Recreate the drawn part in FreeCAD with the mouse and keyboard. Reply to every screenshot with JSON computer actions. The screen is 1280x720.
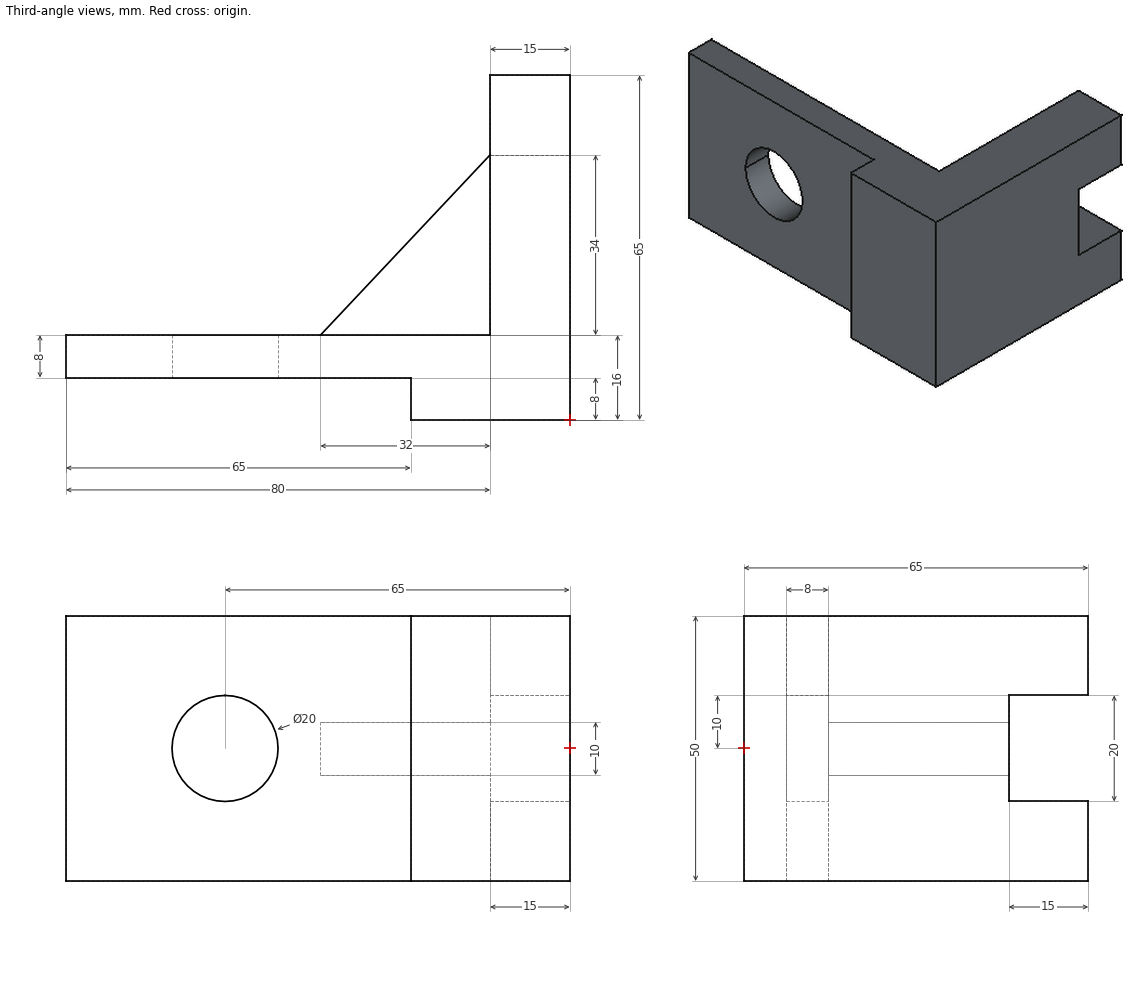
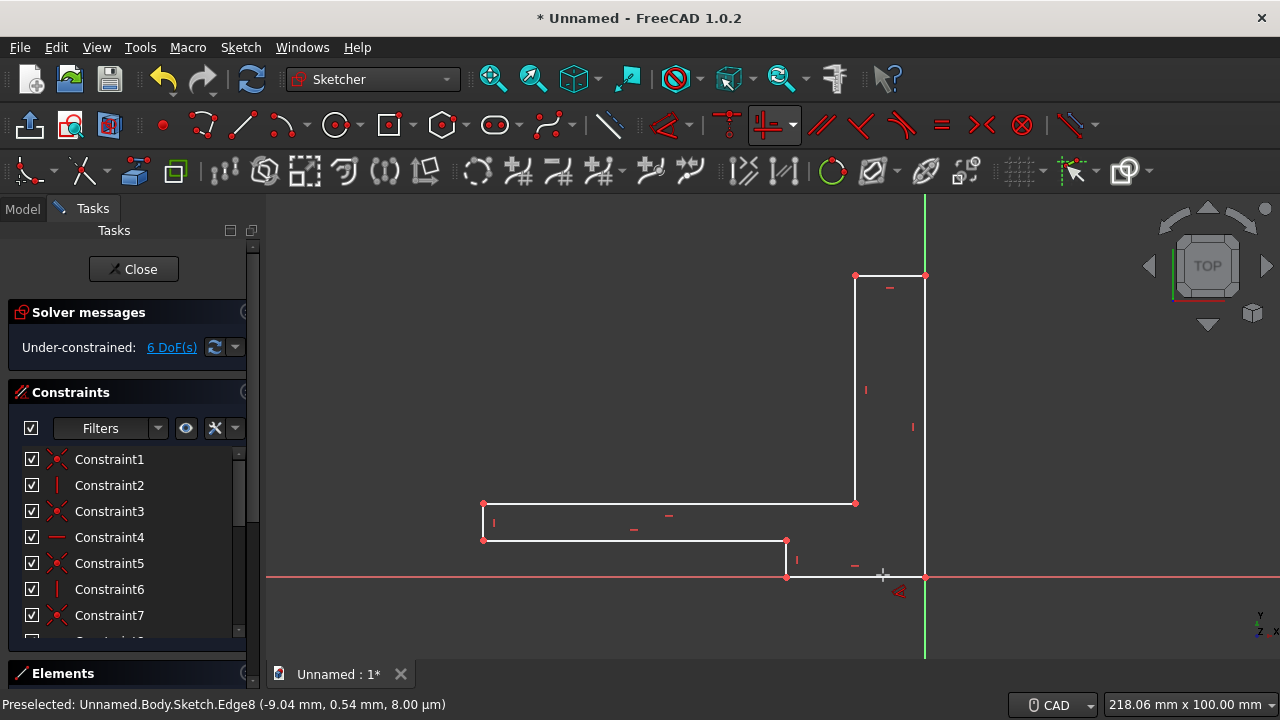
{"action": "scroll", "coordinate": [483, 515], "scroll_direction": "up", "scroll_amount": 2}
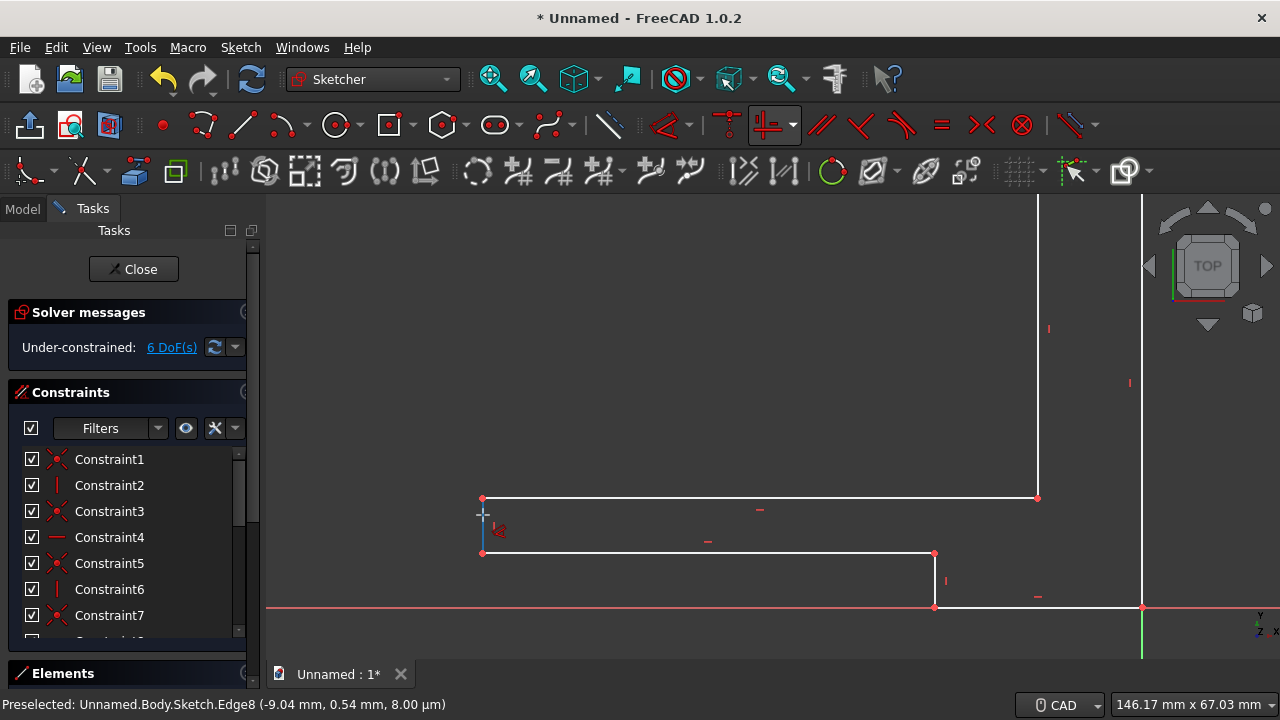
{"action": "left_click", "coordinate": [483, 515]}
{"action": "left_click", "coordinate": [449, 526]}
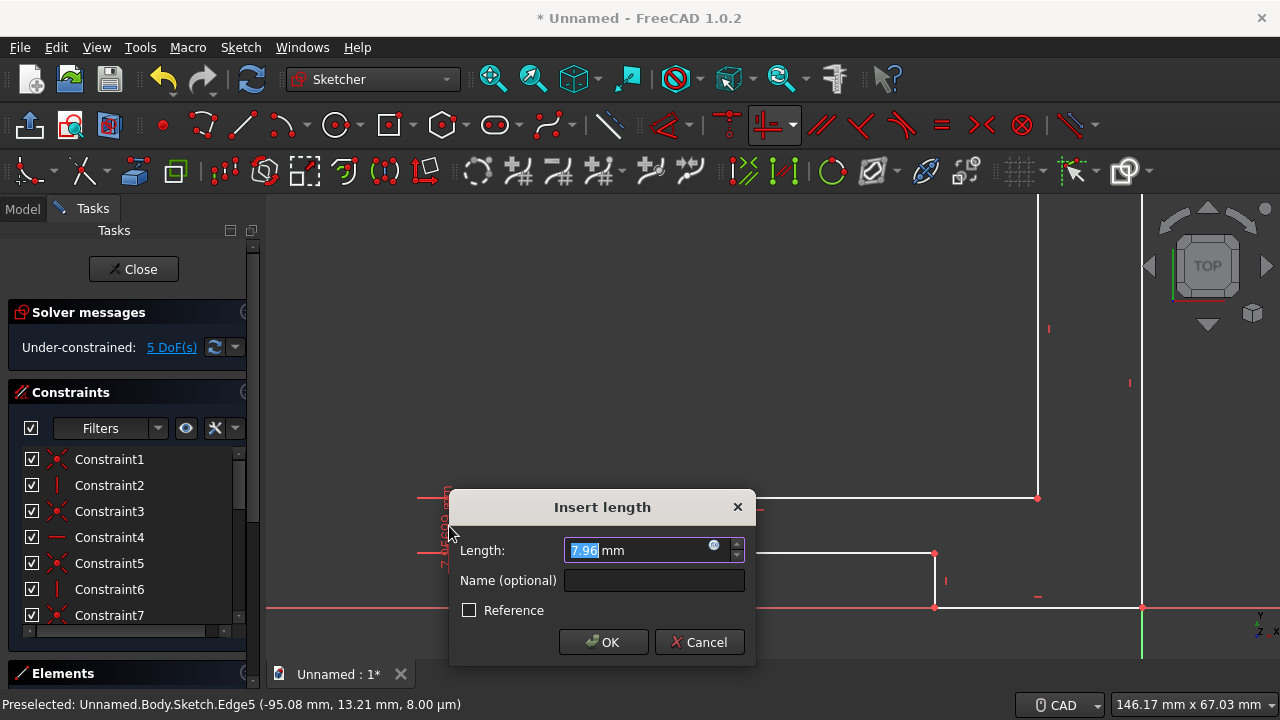
{"action": "type", "text": "8"}
{"action": "key", "text": "Return"}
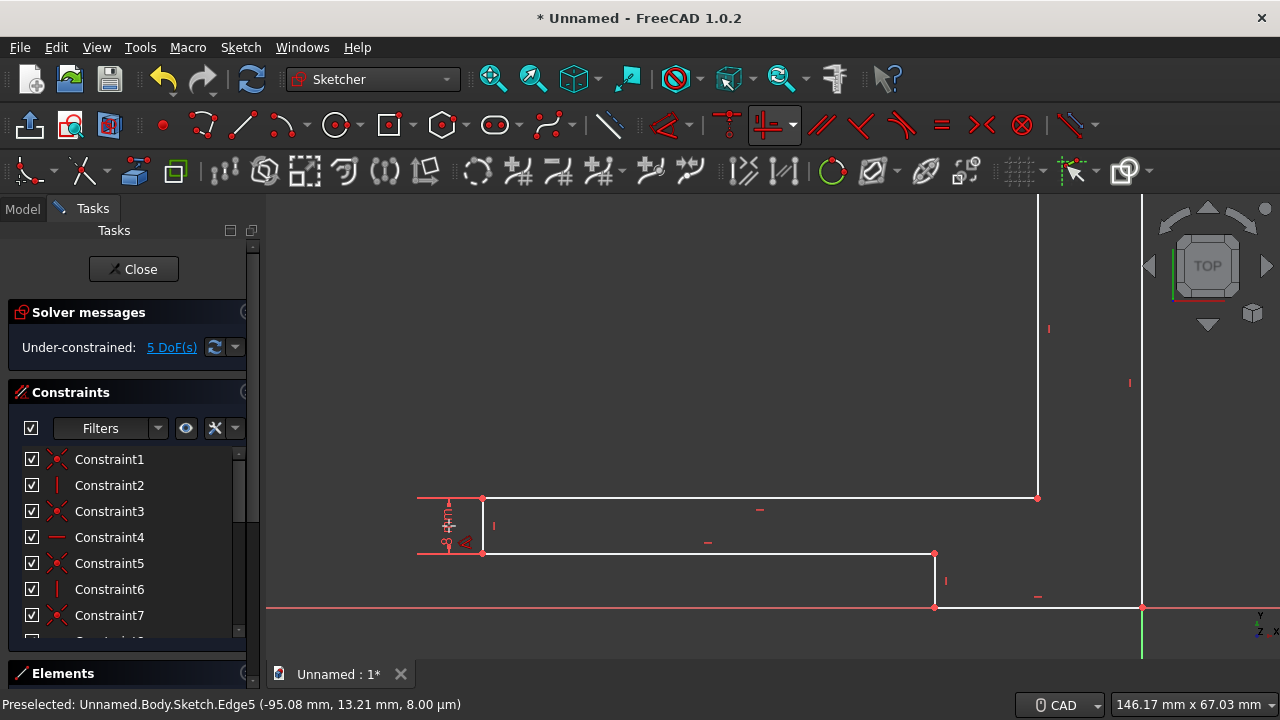
{"action": "left_click", "coordinate": [935, 570]}
{"action": "left_click", "coordinate": [969, 581]}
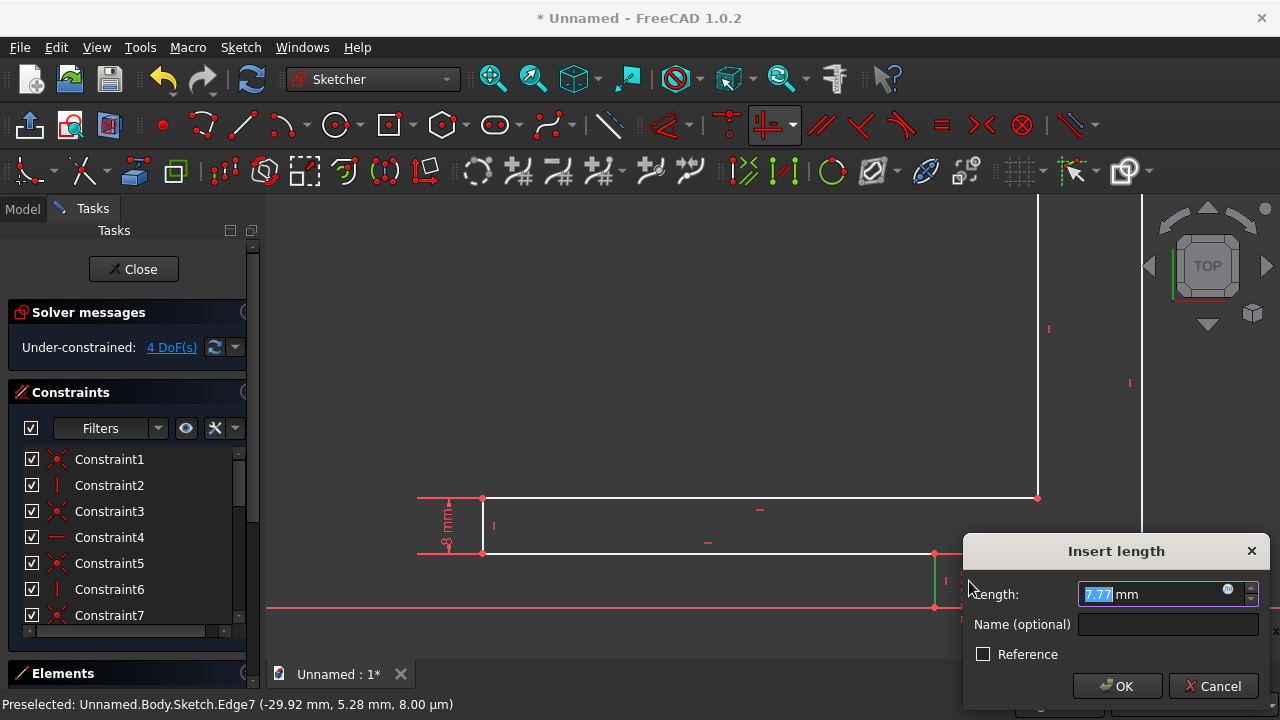
{"action": "type", "text": "8"}
{"action": "key", "text": "Return"}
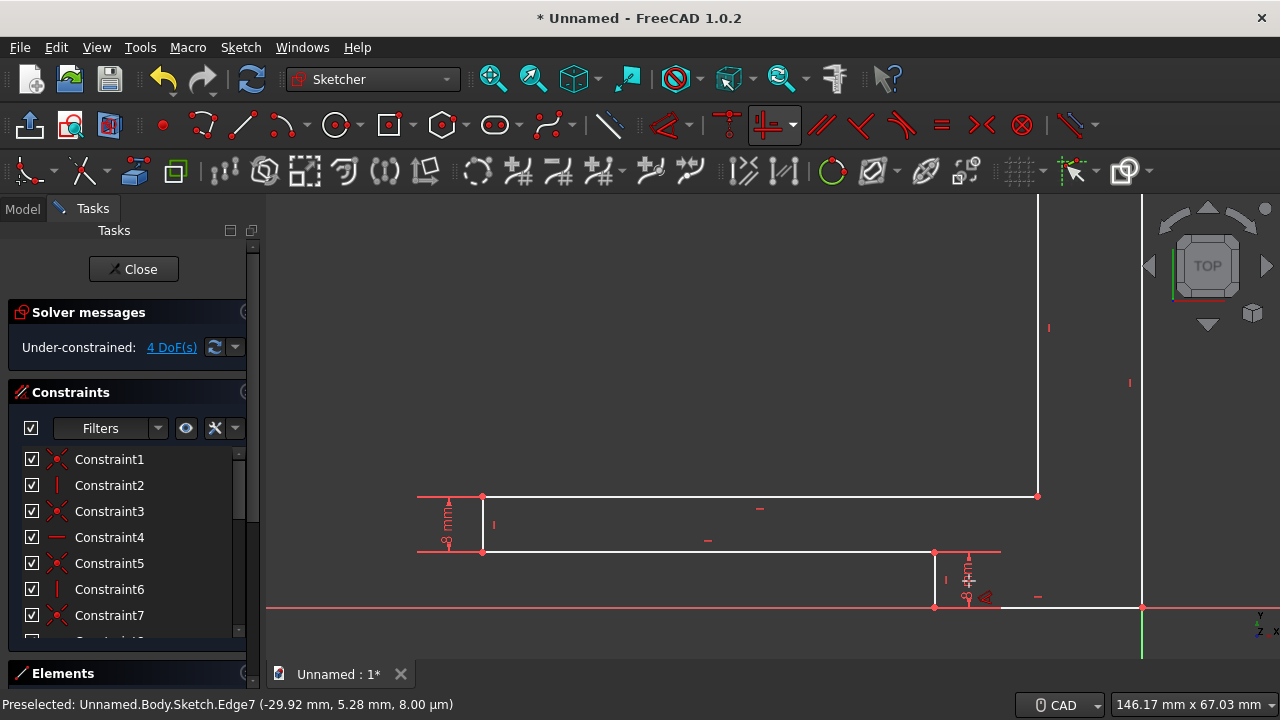
{"action": "scroll", "coordinate": [484, 517], "scroll_direction": "down", "scroll_amount": 2}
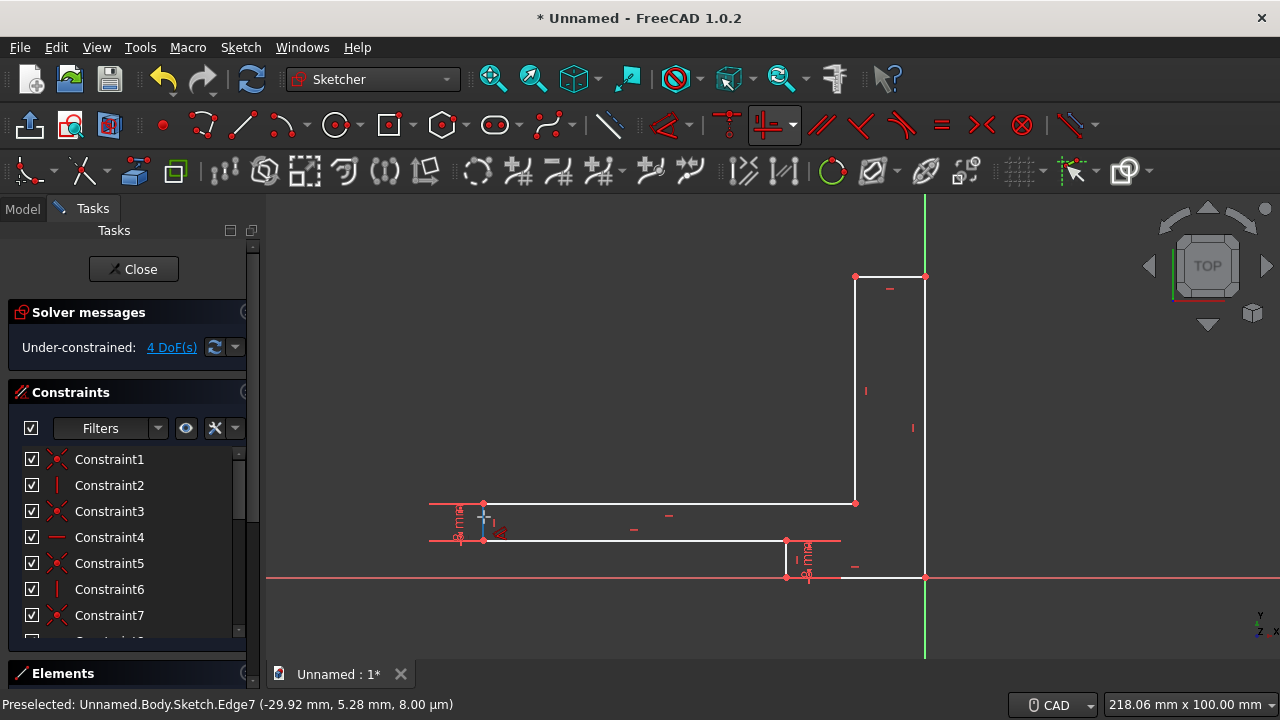
{"action": "left_click", "coordinate": [925, 488]}
{"action": "left_click", "coordinate": [959, 427]}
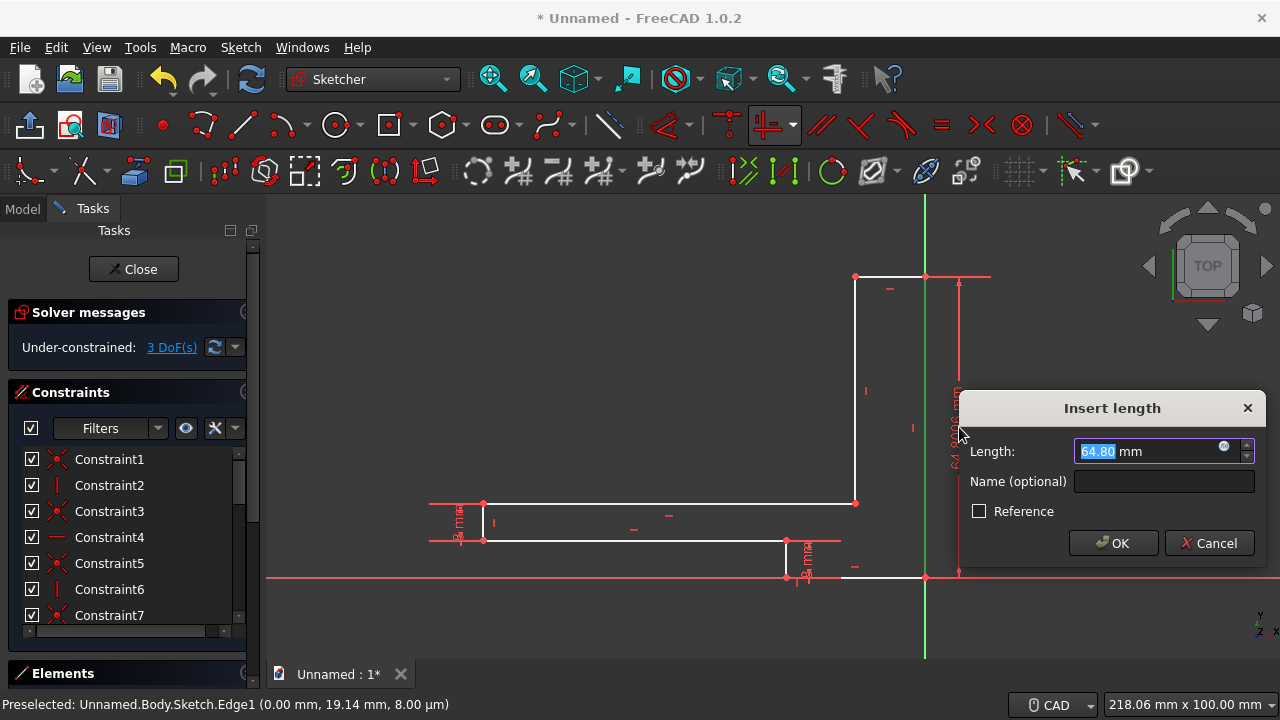
{"action": "type", "text": "65"}
{"action": "key", "text": "Return"}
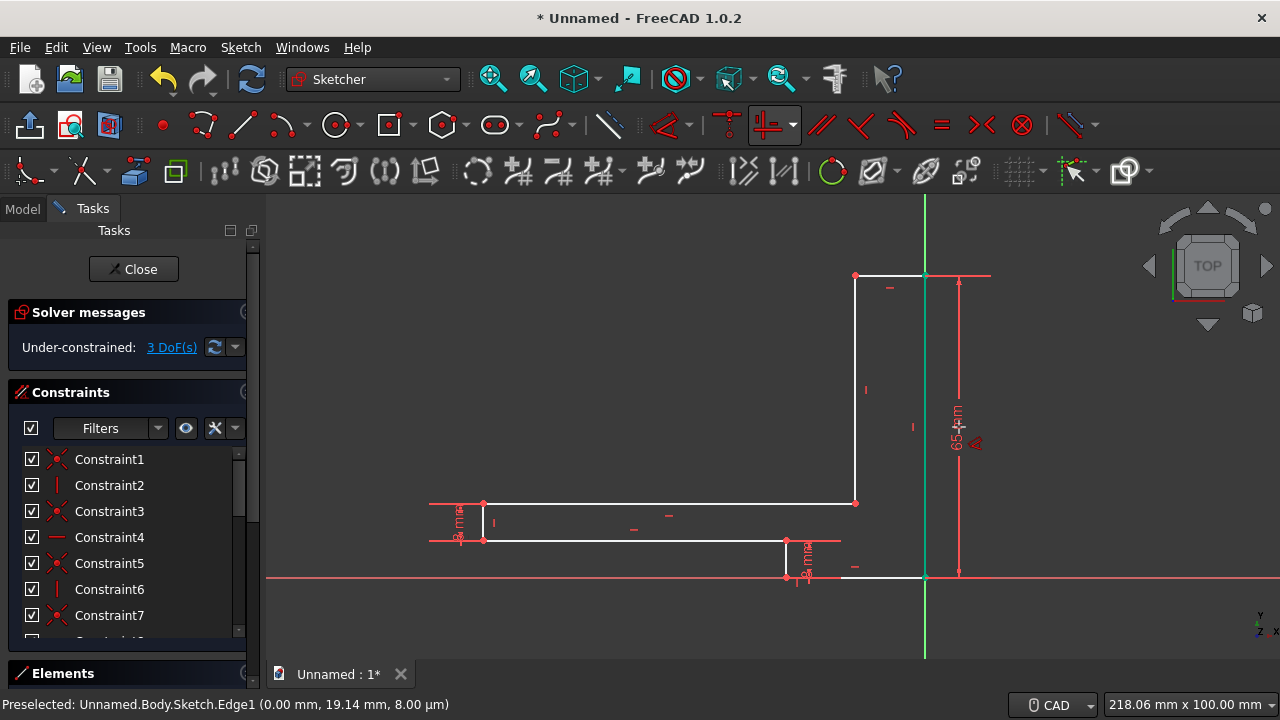
{"action": "left_click", "coordinate": [904, 276]}
{"action": "left_click", "coordinate": [890, 242]}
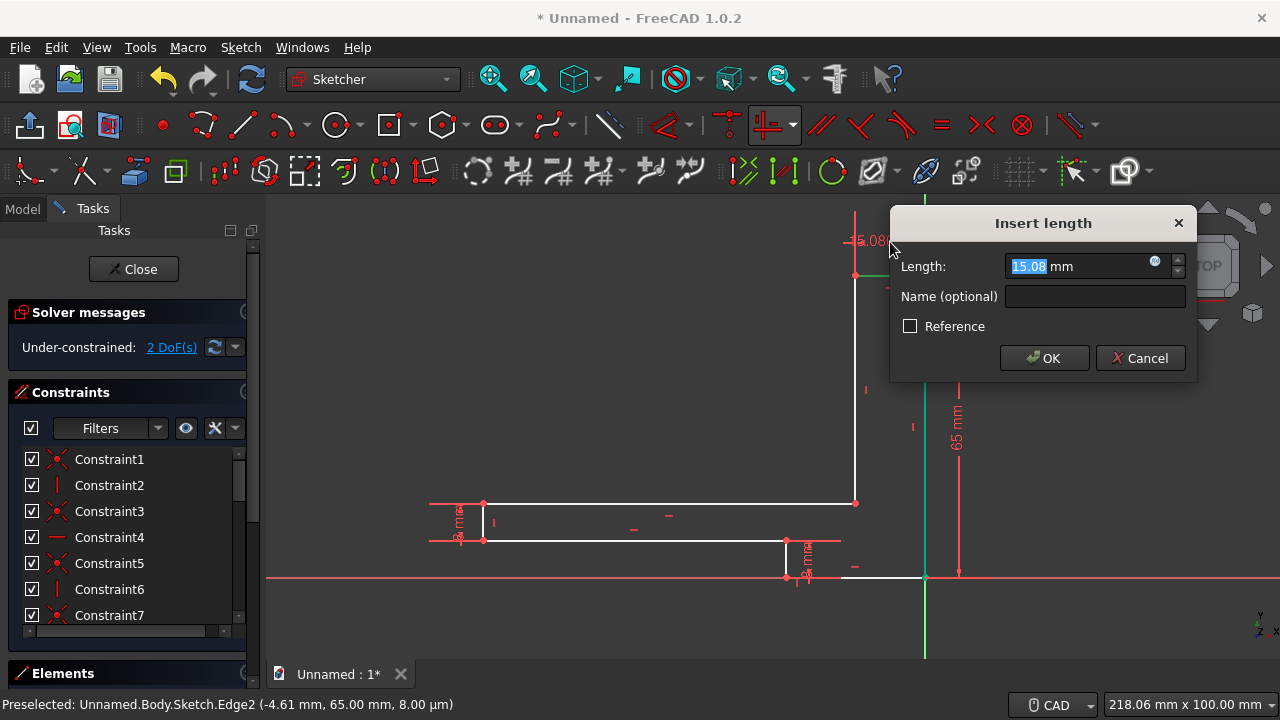
{"action": "type", "text": "15"}
{"action": "key", "text": "Return"}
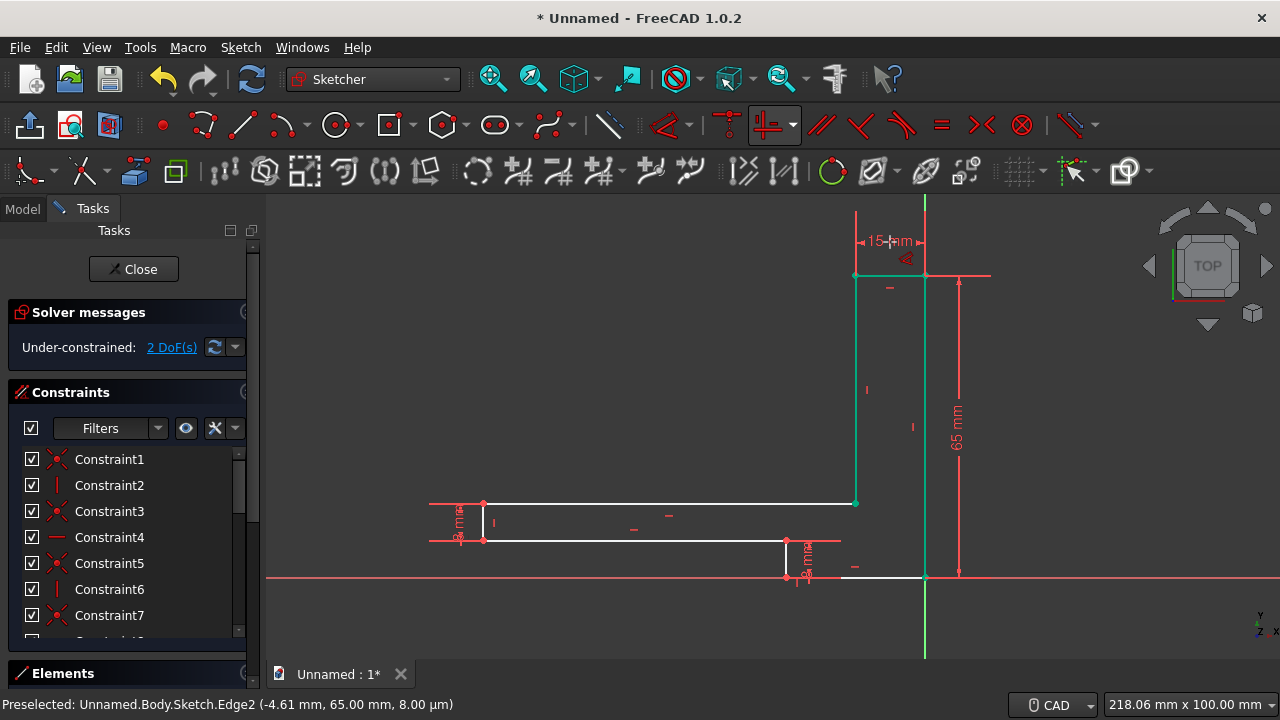
{"action": "left_click", "coordinate": [744, 504]}
{"action": "left_click", "coordinate": [800, 538]}